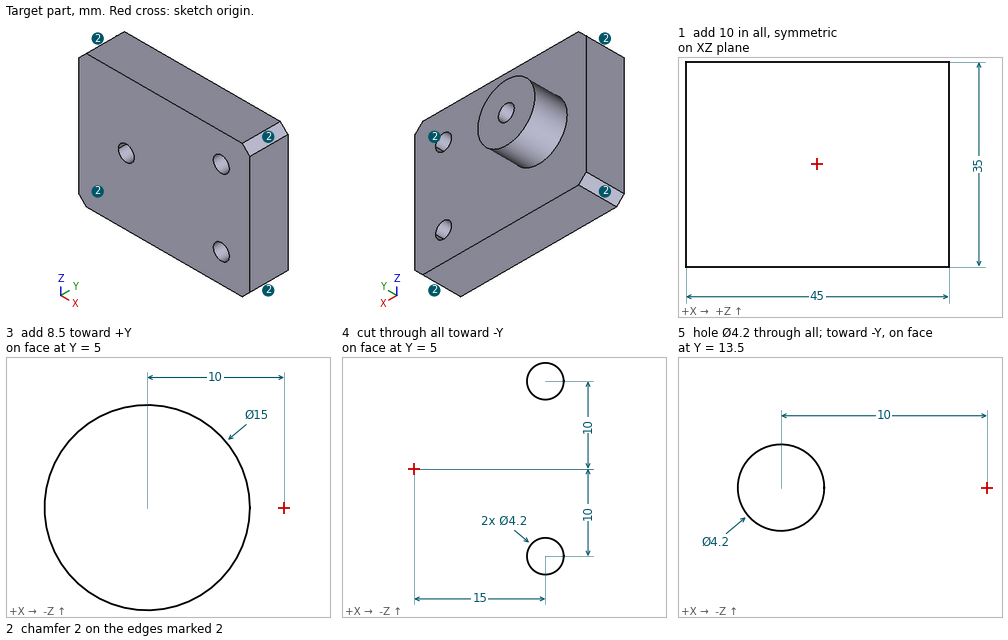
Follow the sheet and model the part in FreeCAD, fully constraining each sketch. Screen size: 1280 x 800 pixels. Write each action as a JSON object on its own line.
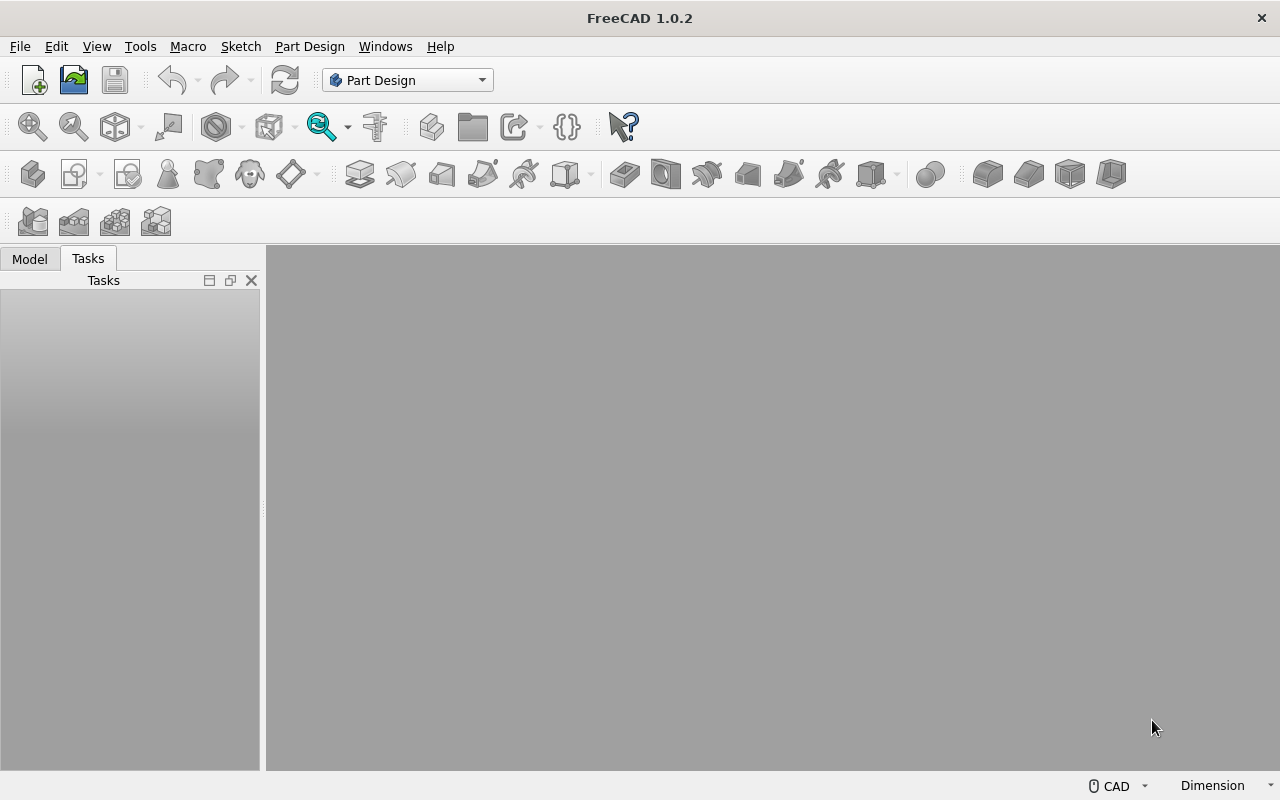
{"action": "left_click", "coordinate": [33, 80]}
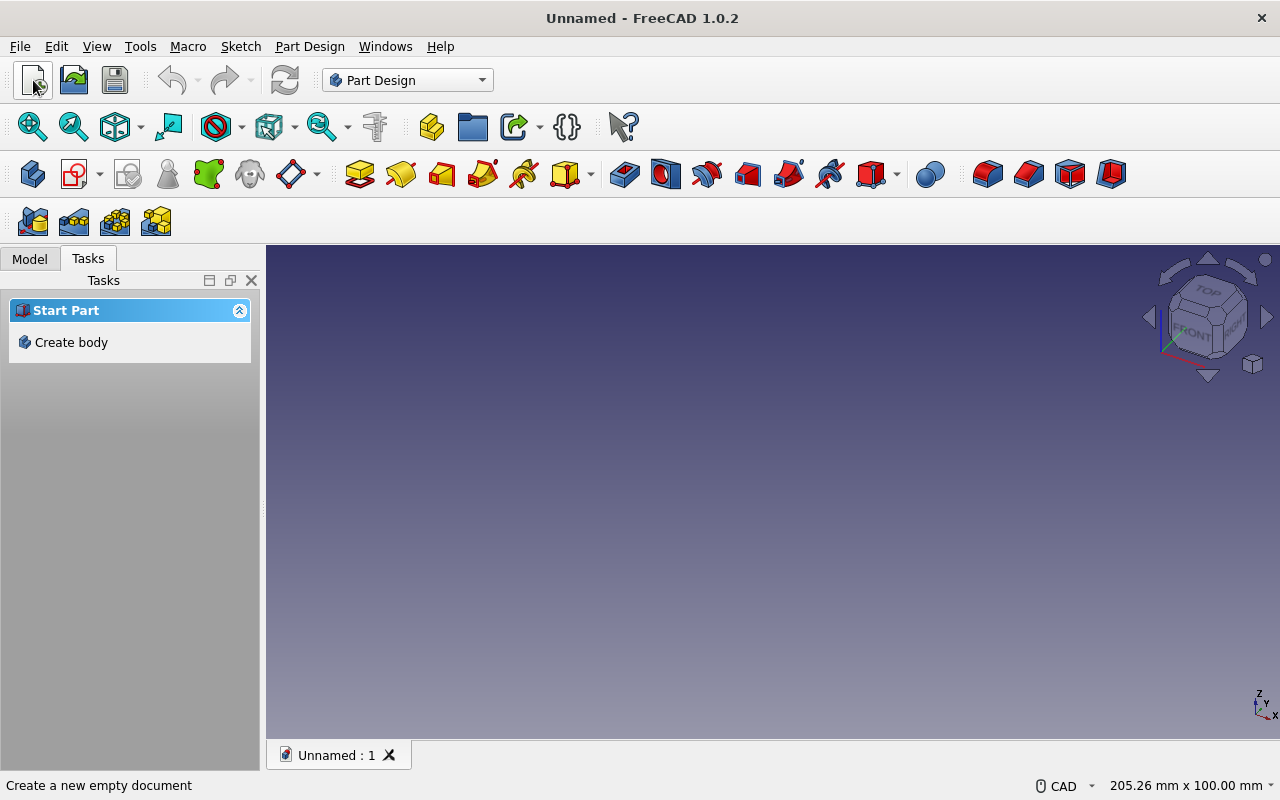
{"action": "left_click", "coordinate": [74, 174]}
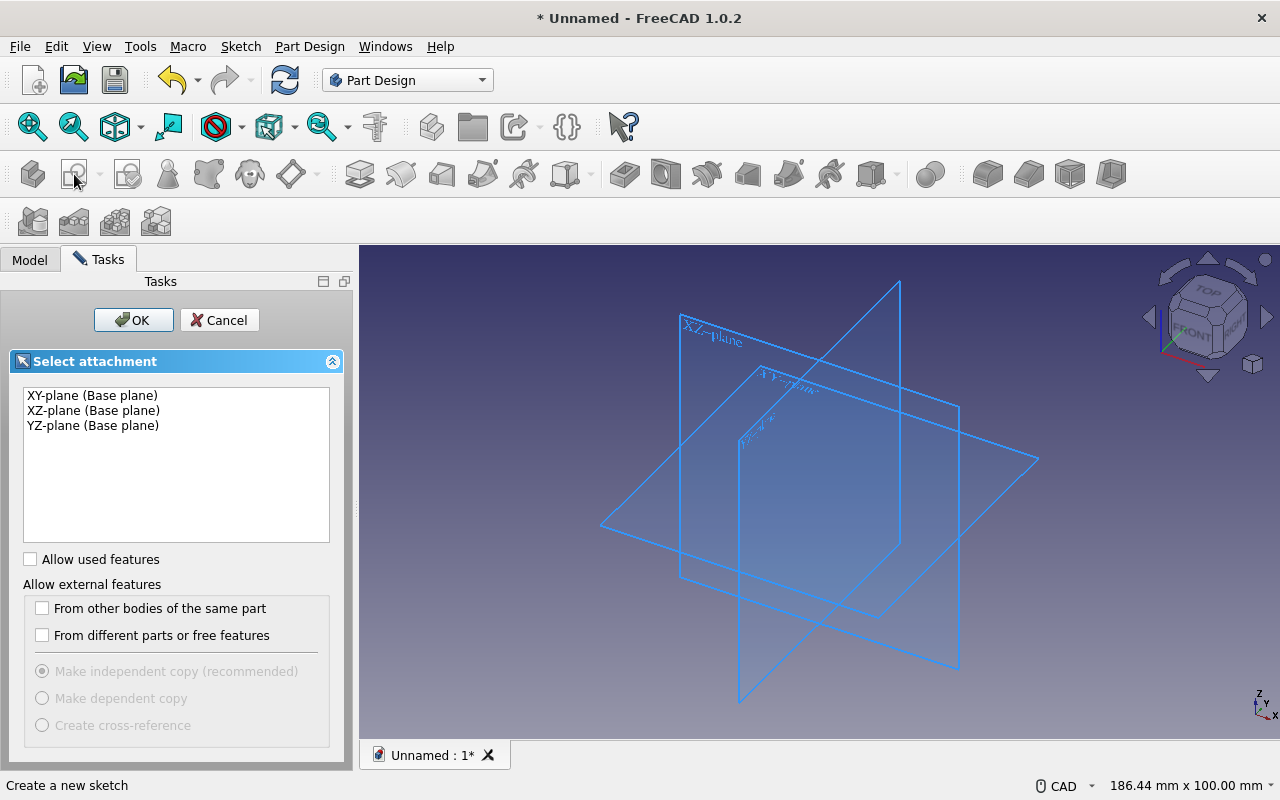
{"action": "left_click", "coordinate": [84, 410]}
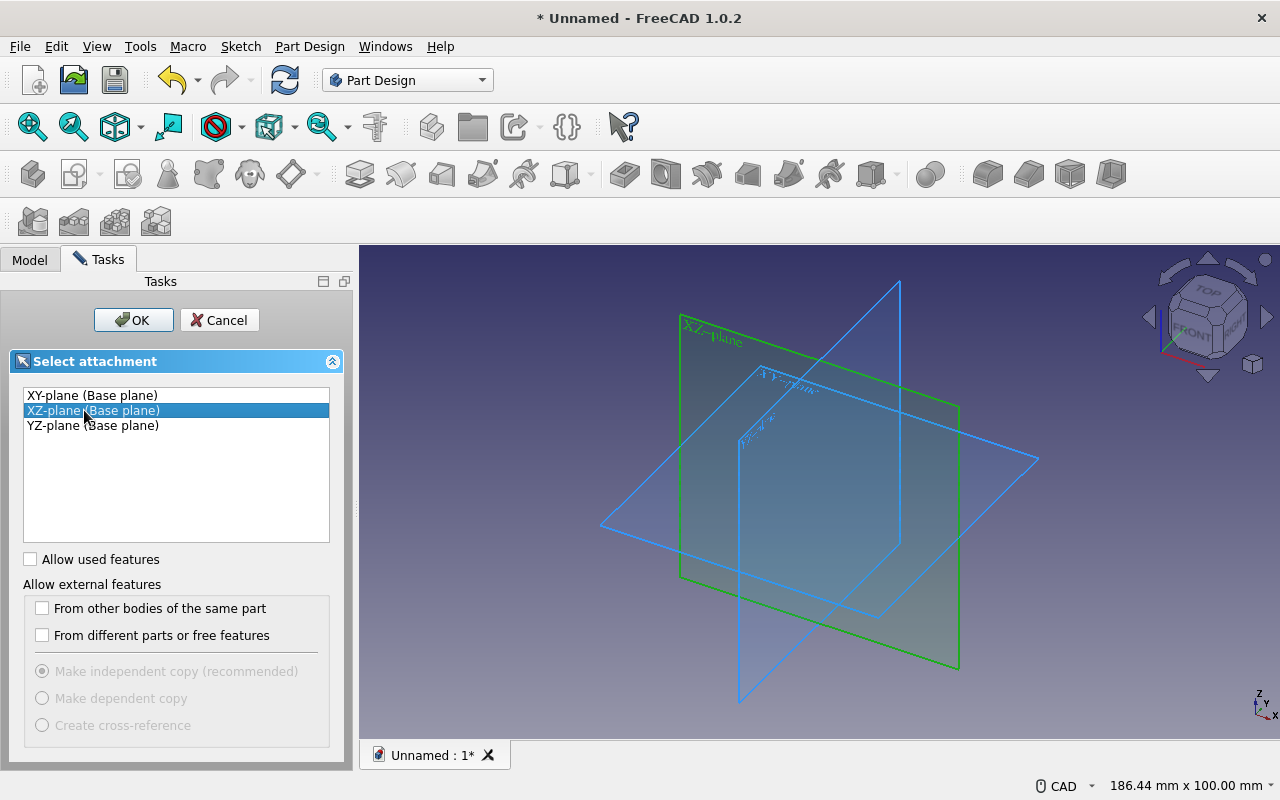
{"action": "left_click", "coordinate": [134, 320]}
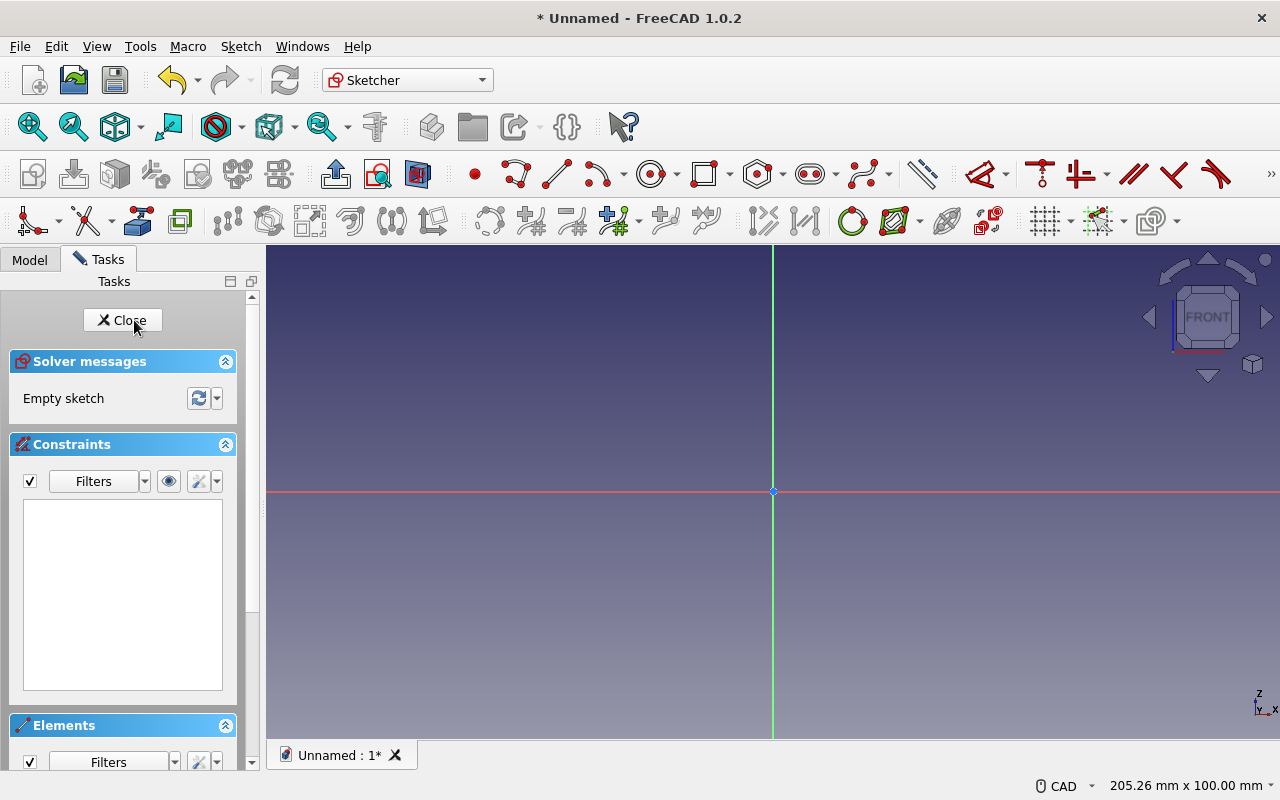
{"action": "scroll", "coordinate": [856, 492], "scroll_direction": "up", "scroll_amount": 3}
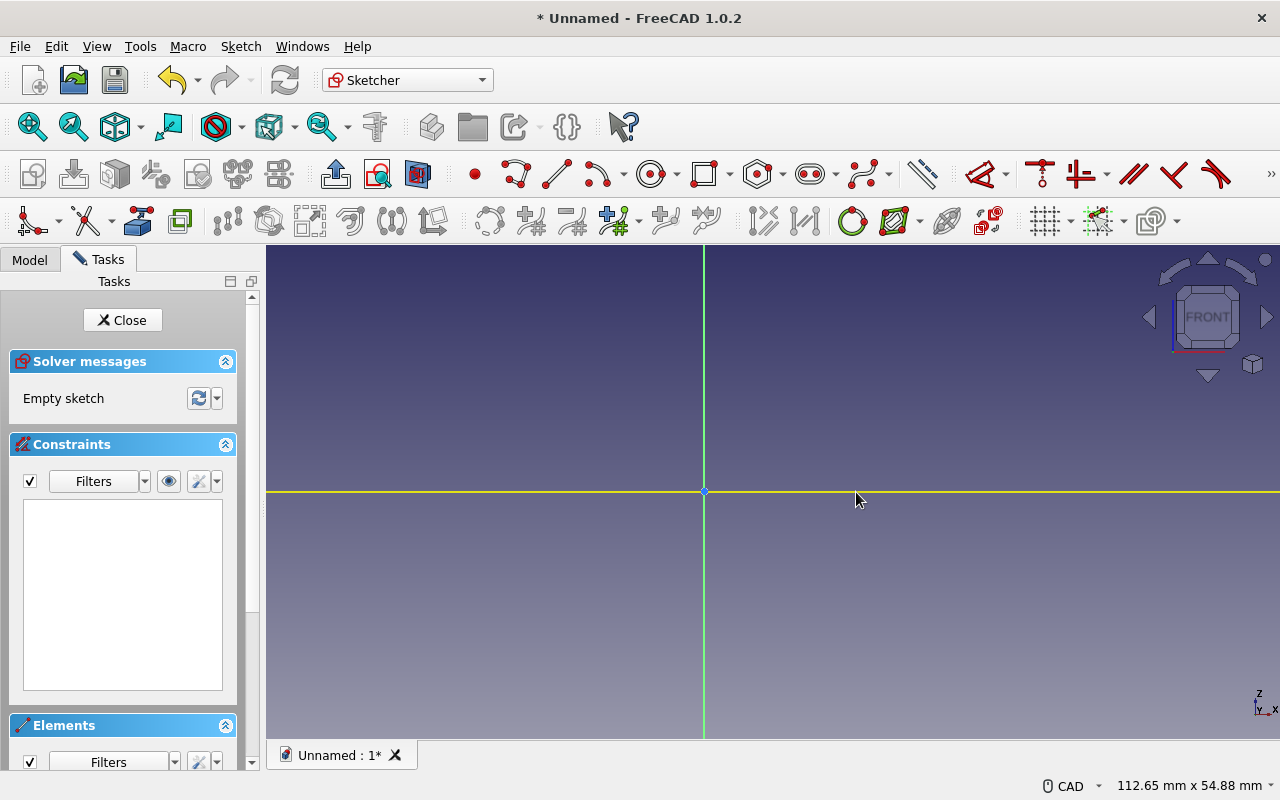
{"action": "key", "text": "g v"}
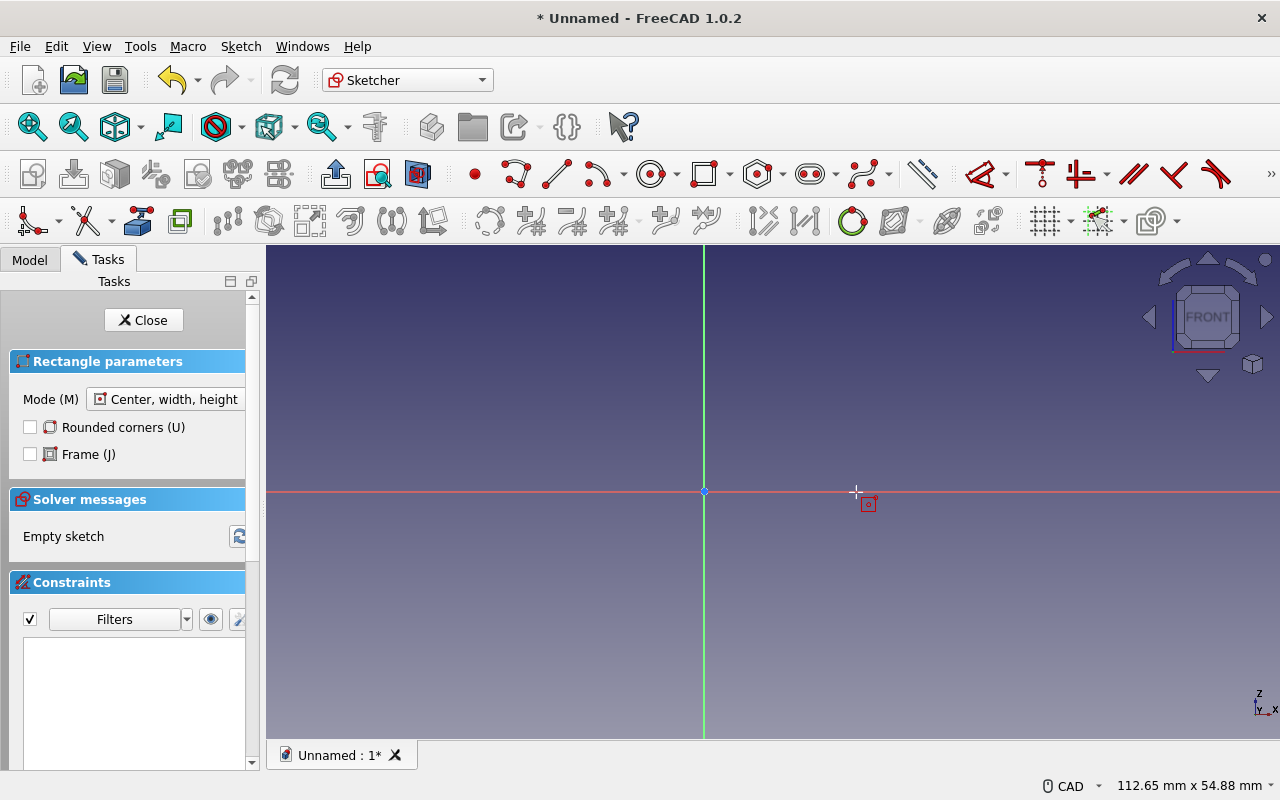
{"action": "left_click", "coordinate": [704, 492]}
{"action": "mouse_move", "coordinate": [907, 334]}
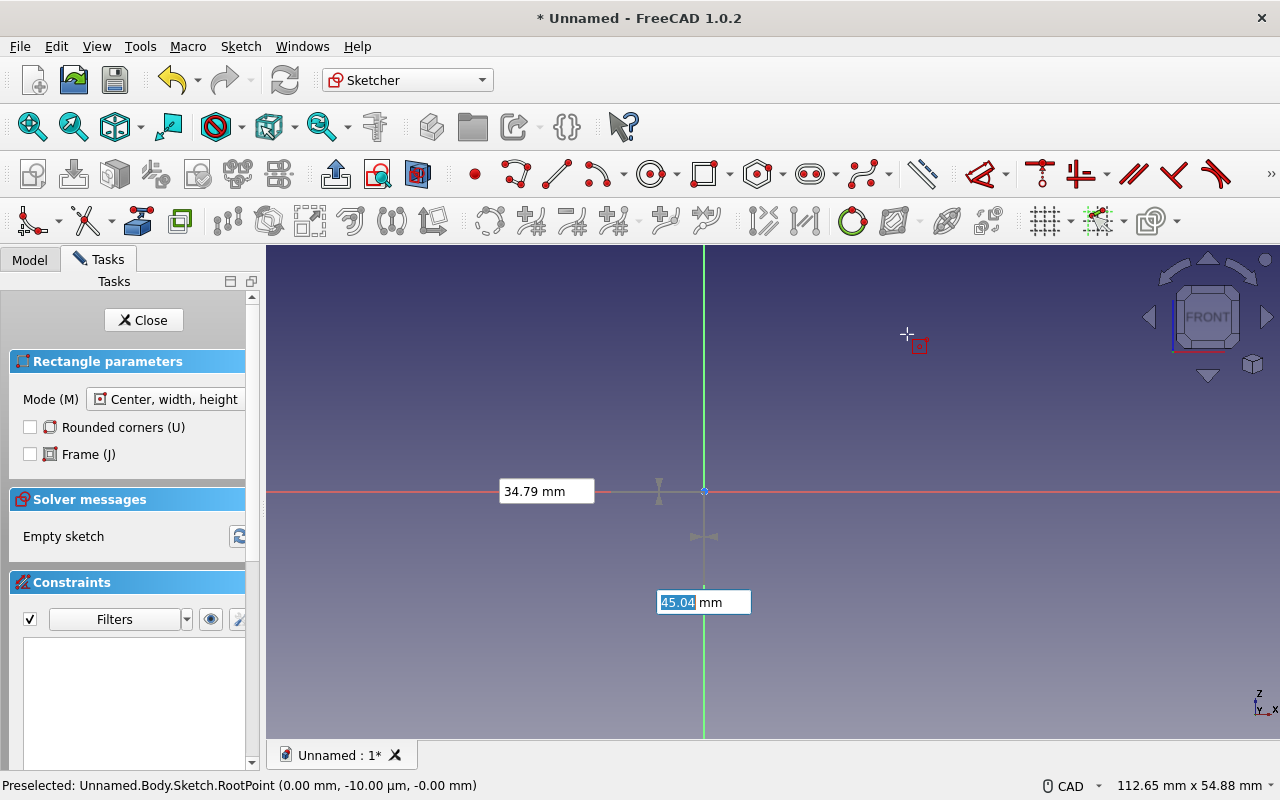
{"action": "type", "text": "45"}
{"action": "key", "text": "Tab"}
{"action": "type", "text": "35"}
{"action": "key", "text": "Return"}
{"action": "key", "text": "Escape"}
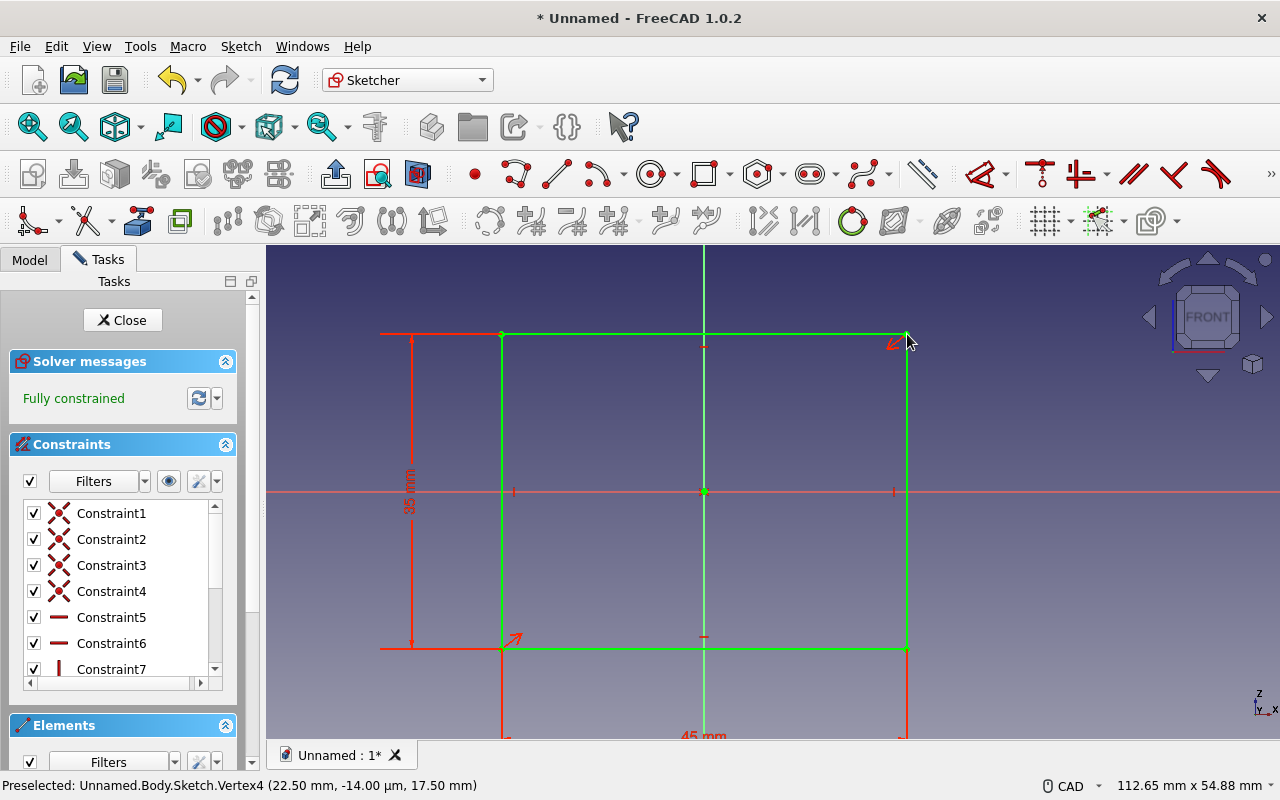
{"action": "left_click", "coordinate": [123, 320]}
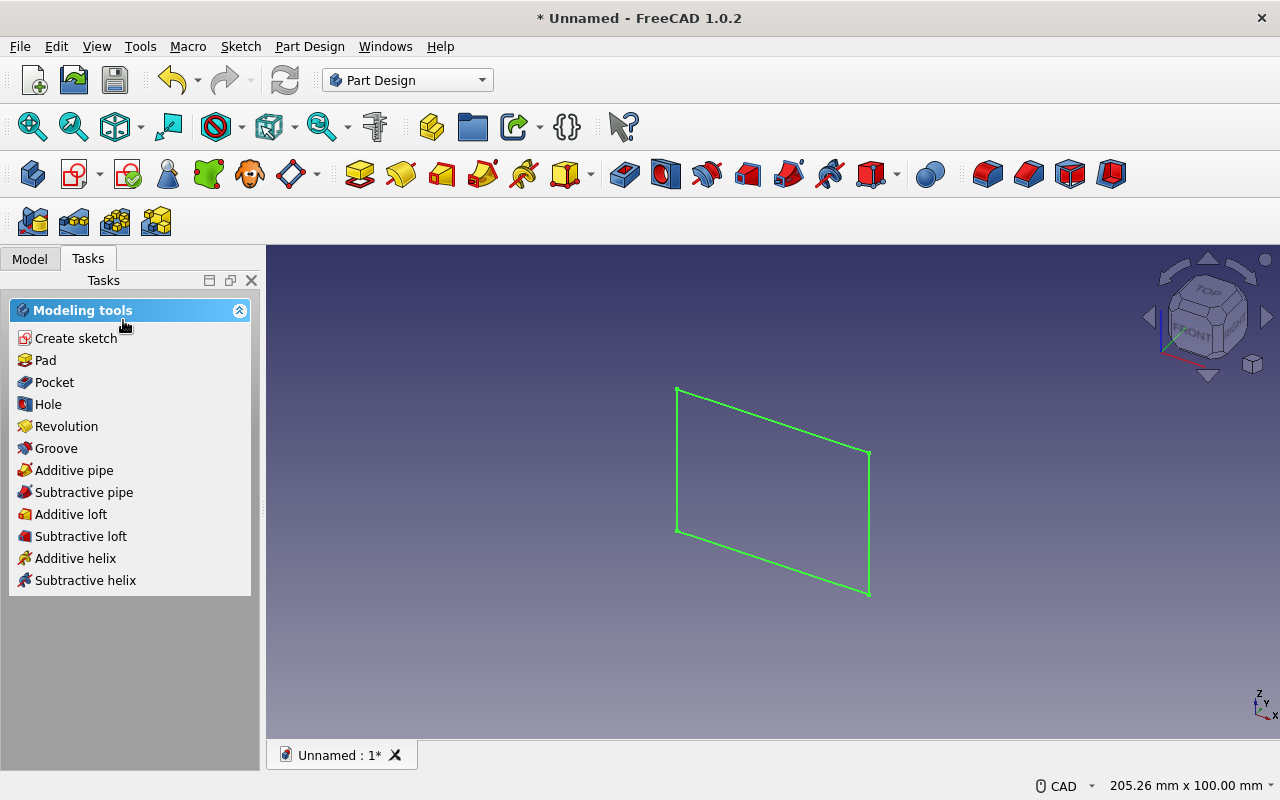
{"action": "left_click", "coordinate": [360, 174]}